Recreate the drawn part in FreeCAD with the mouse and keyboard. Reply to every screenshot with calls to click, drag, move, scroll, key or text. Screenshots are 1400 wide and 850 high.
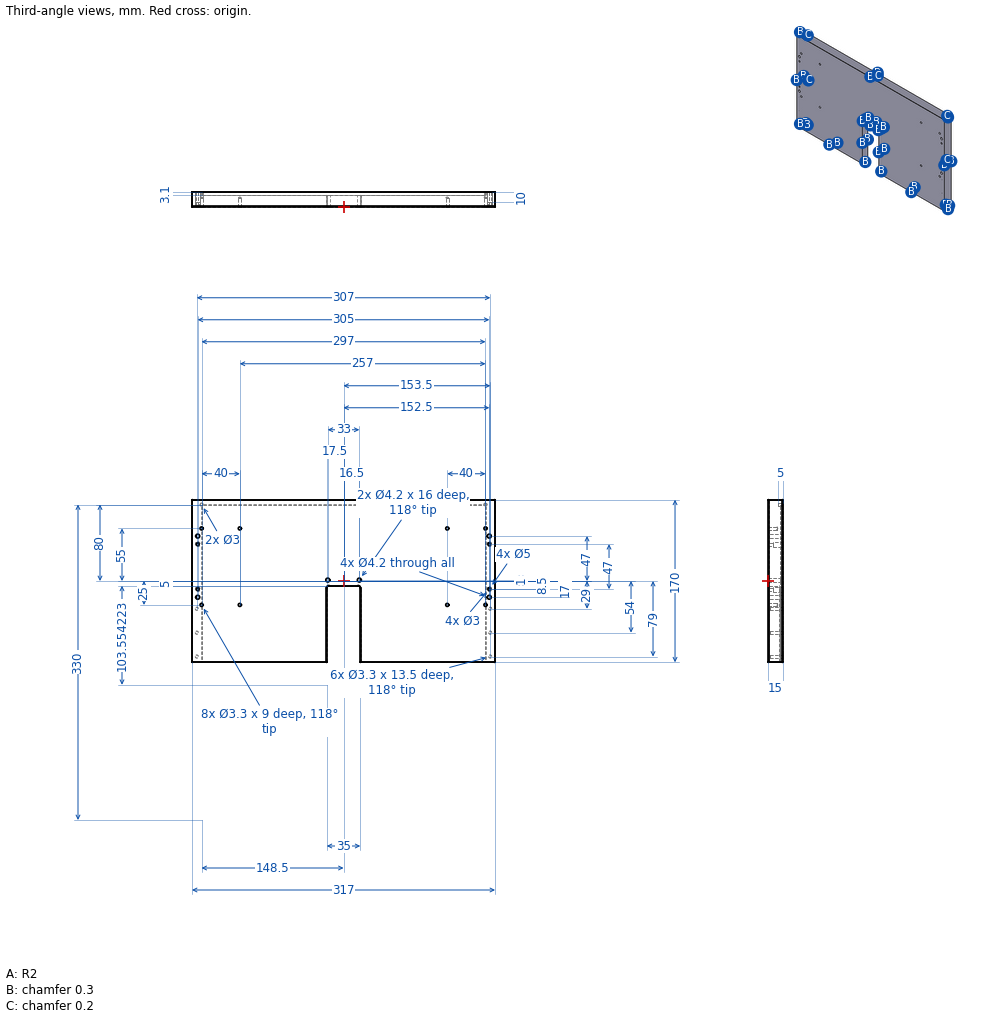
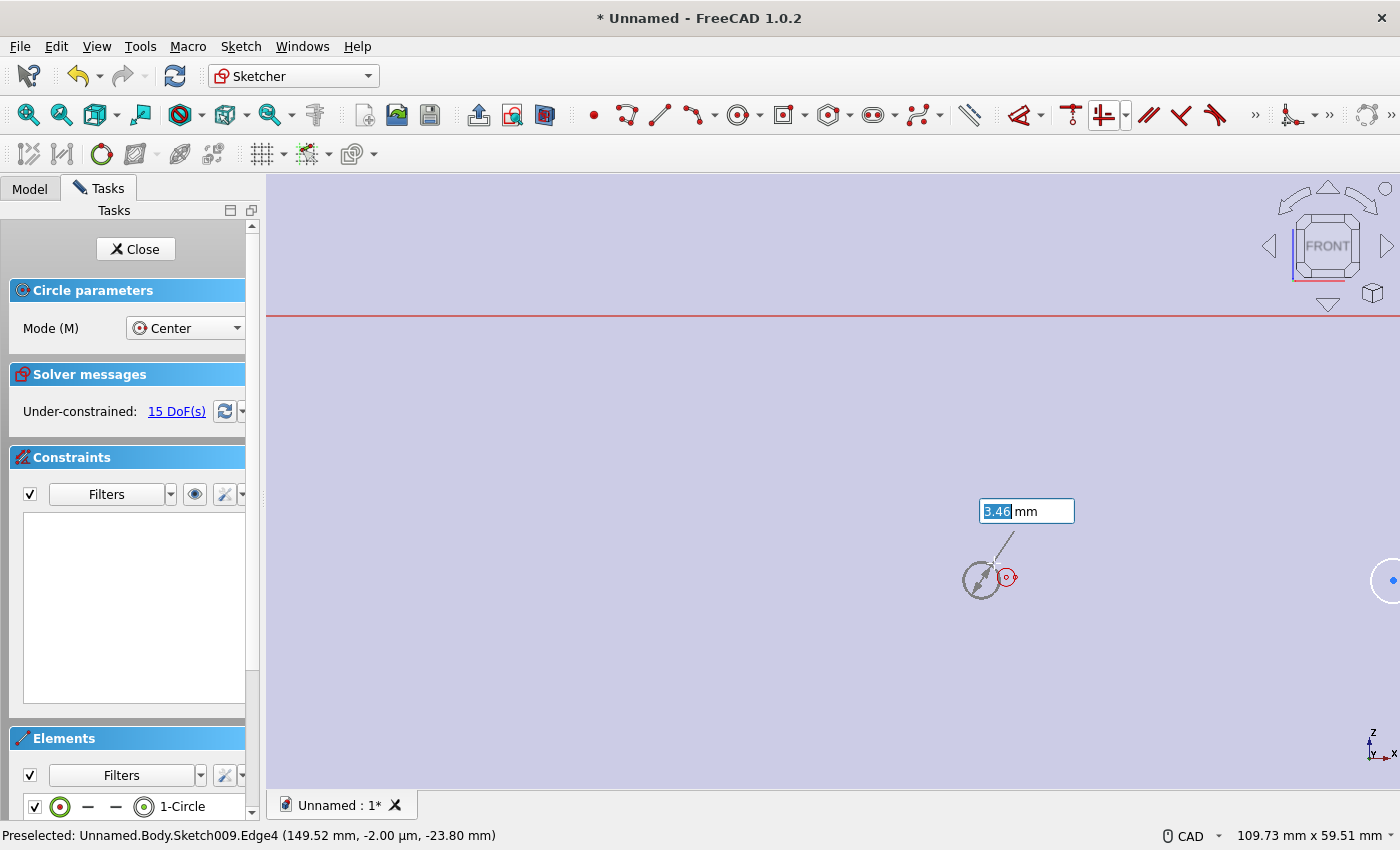
click(993, 563)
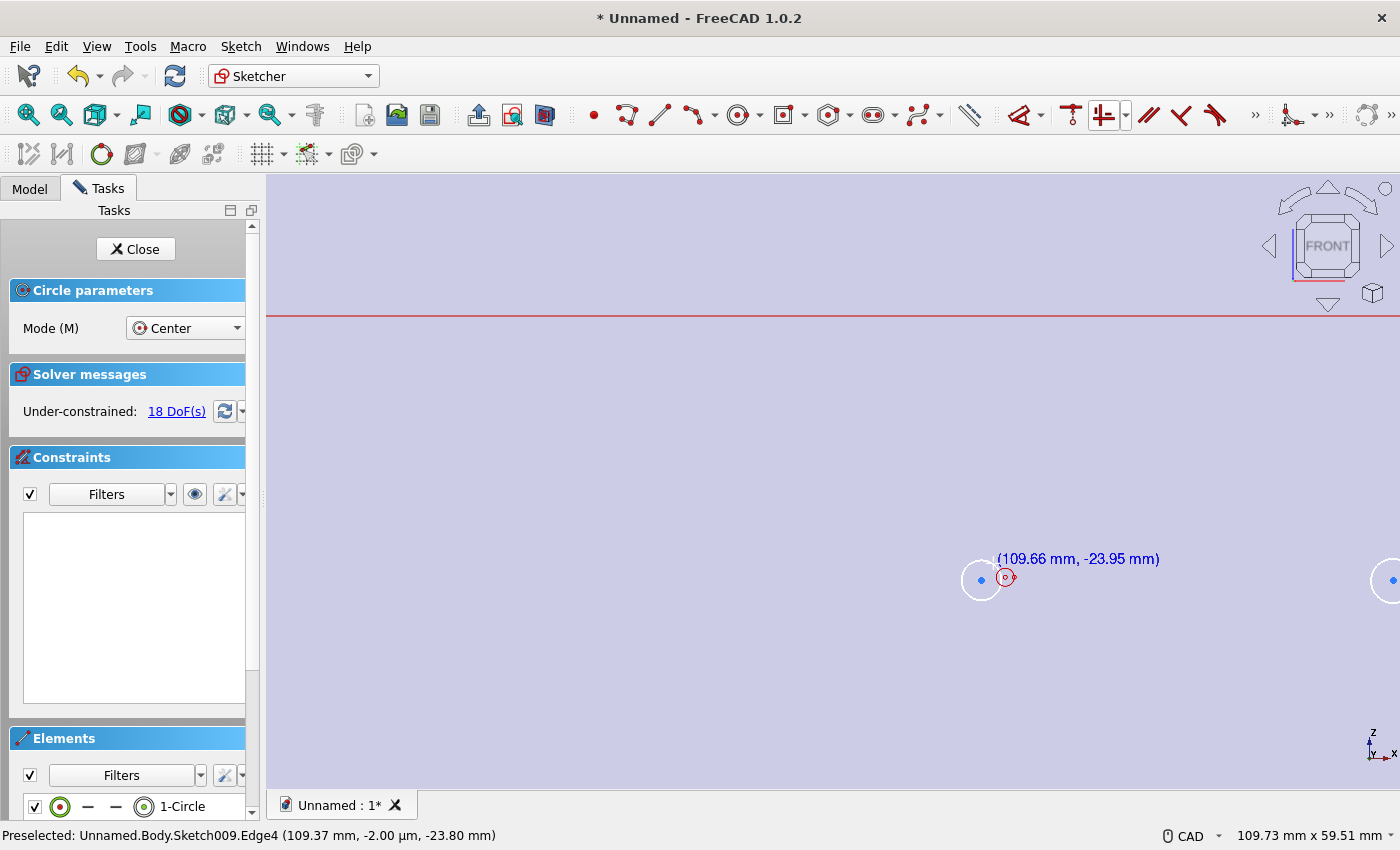
scroll(993, 562, down, 8)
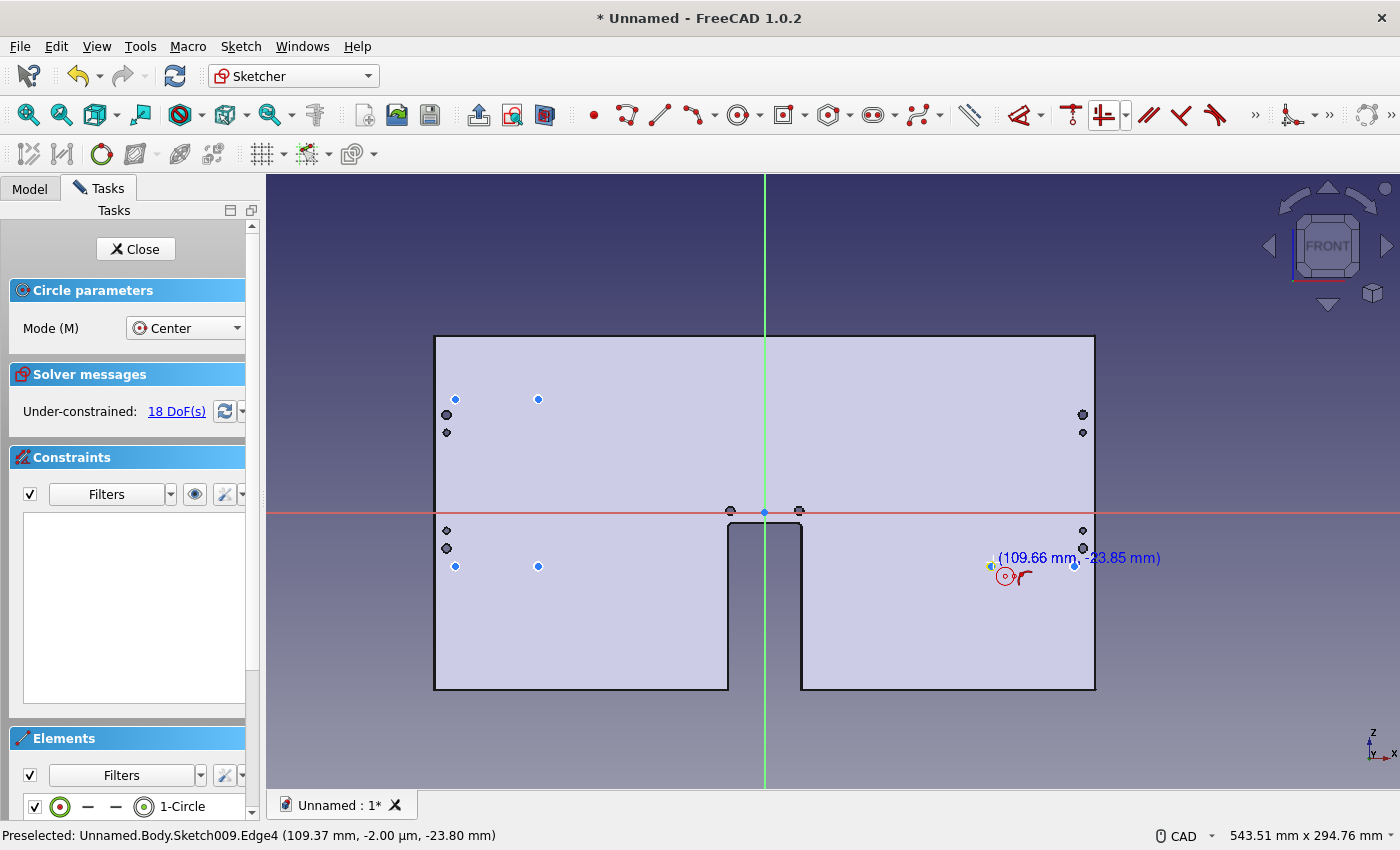
scroll(1075, 398, up, 10)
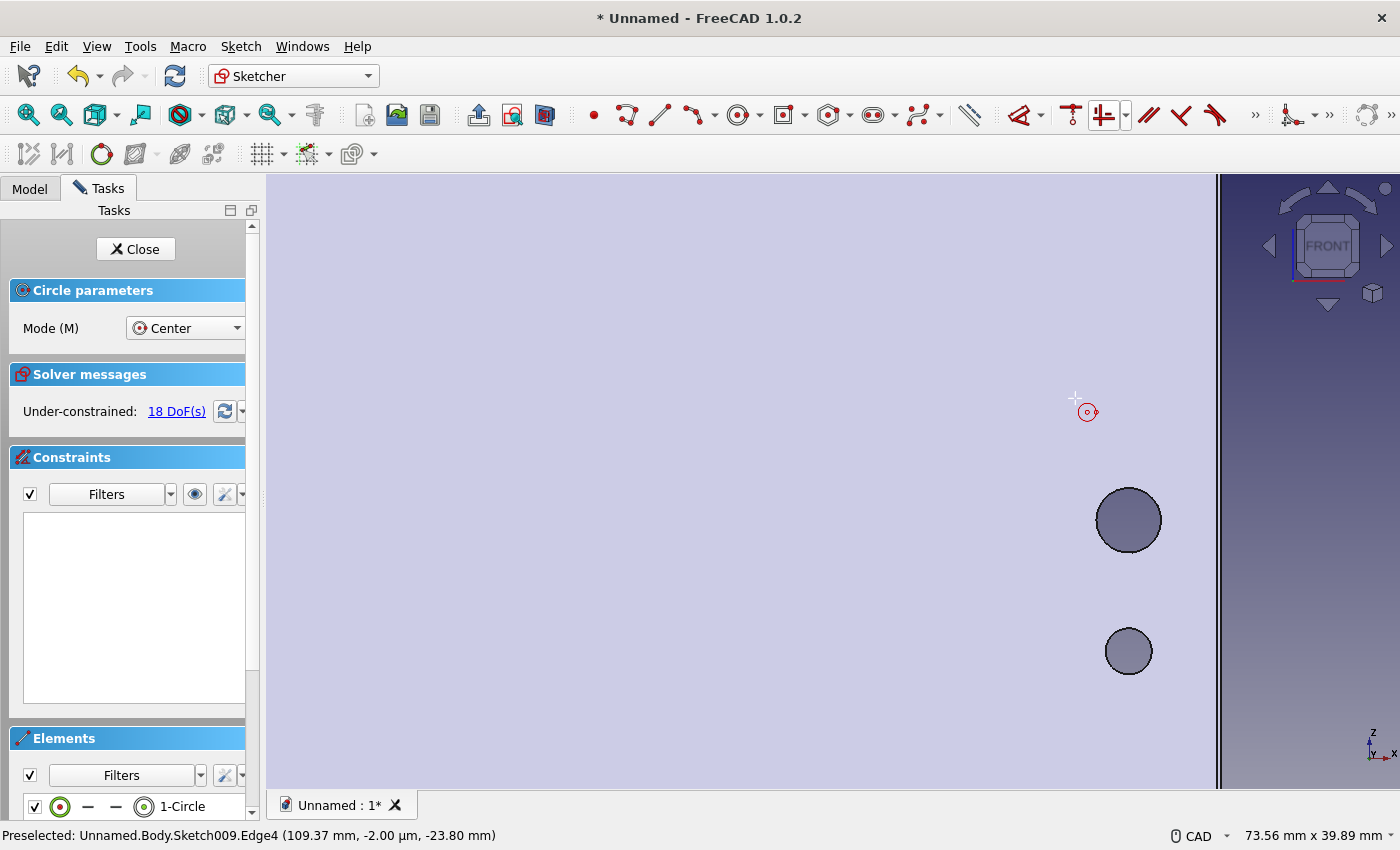
scroll(1075, 398, down, 10)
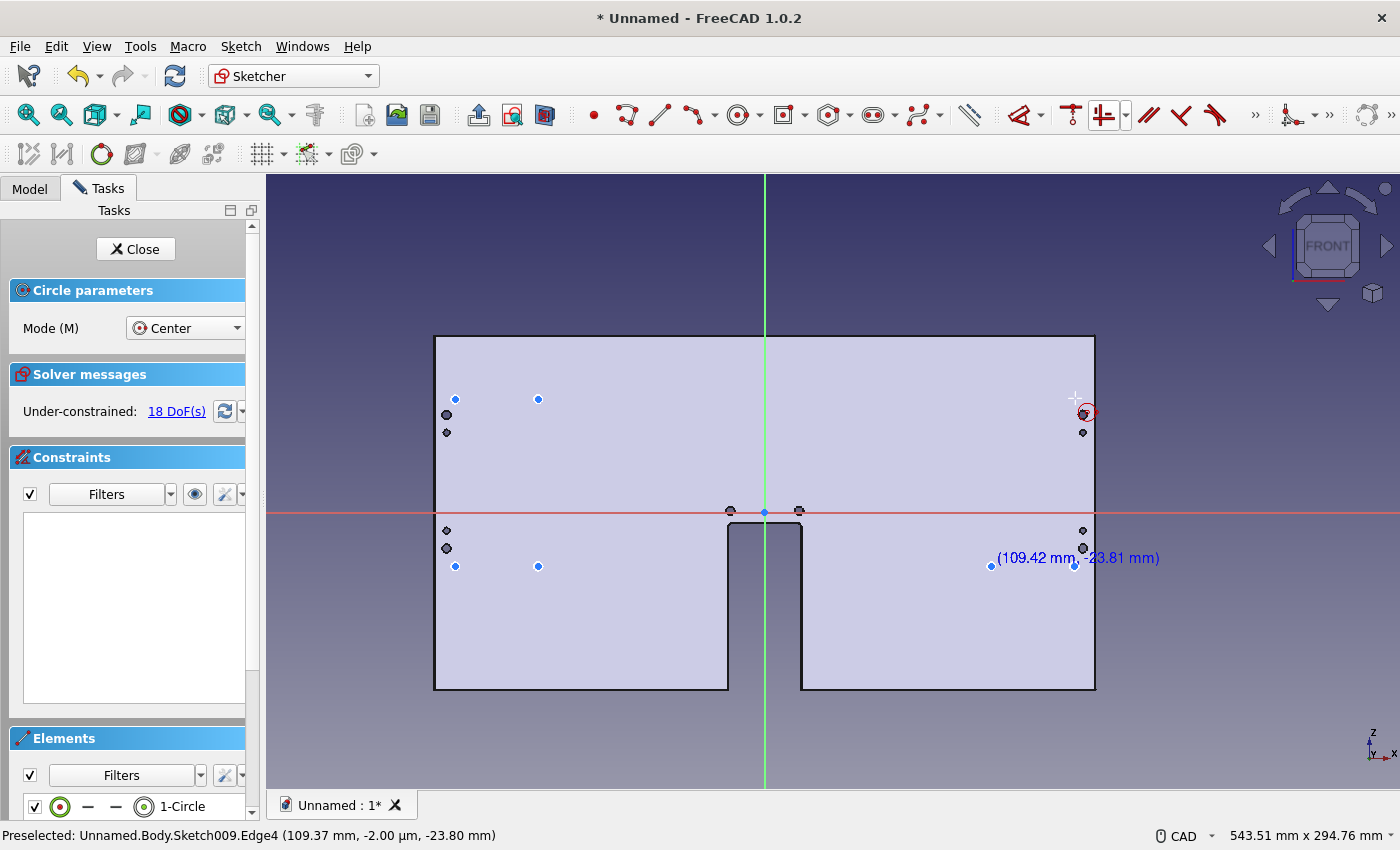
click(1075, 398)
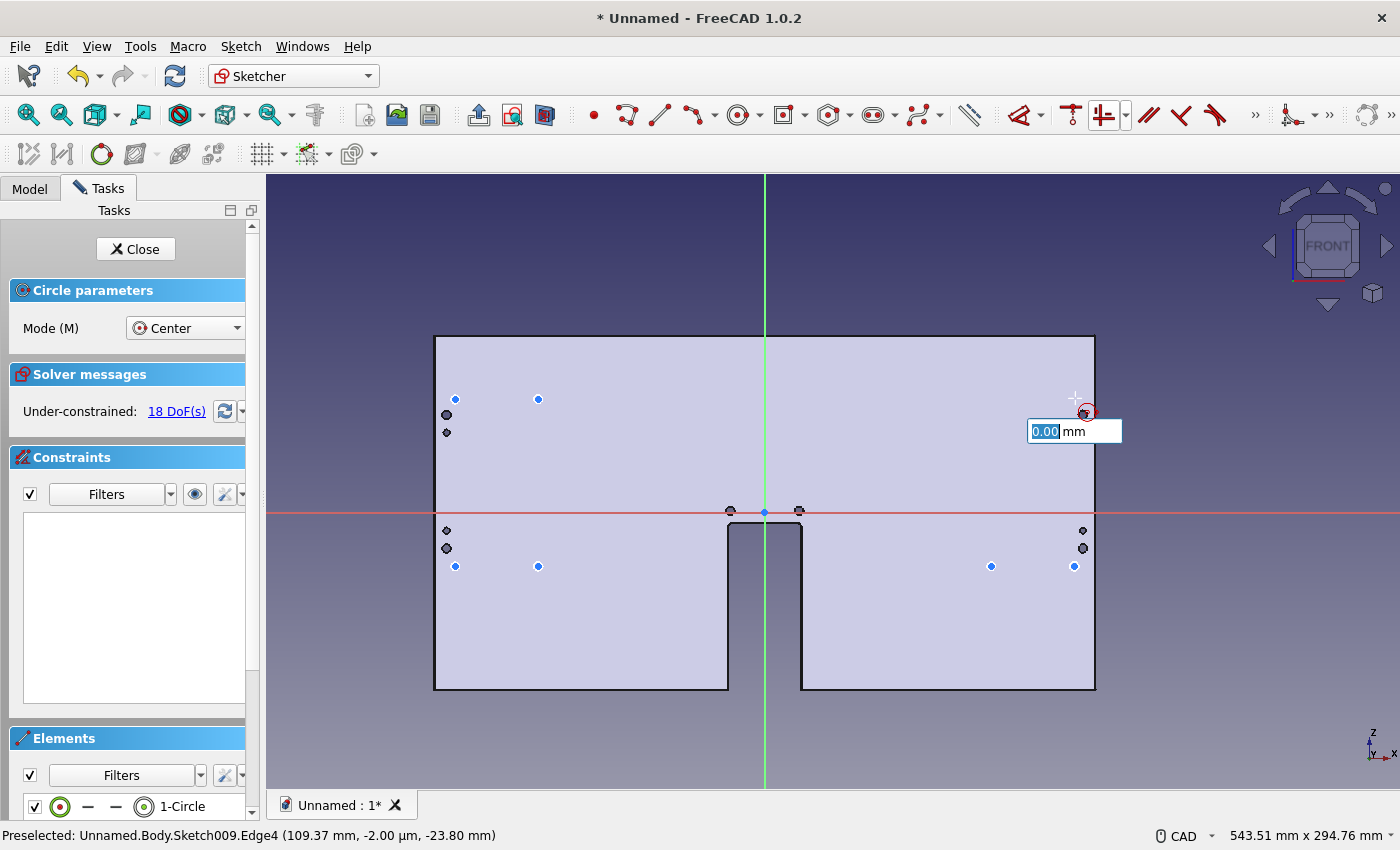
scroll(1077, 396, up, 8)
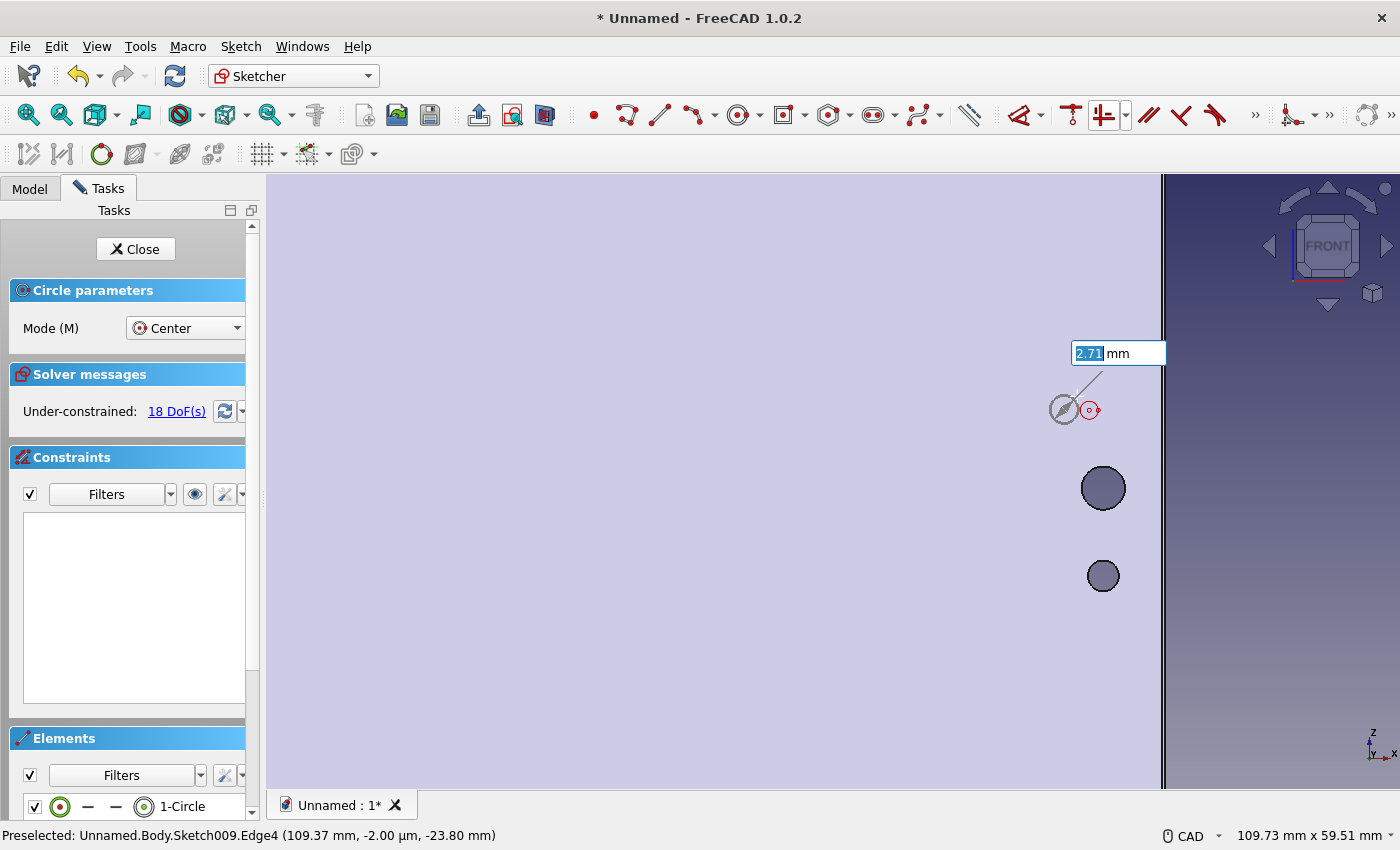
click(1074, 393)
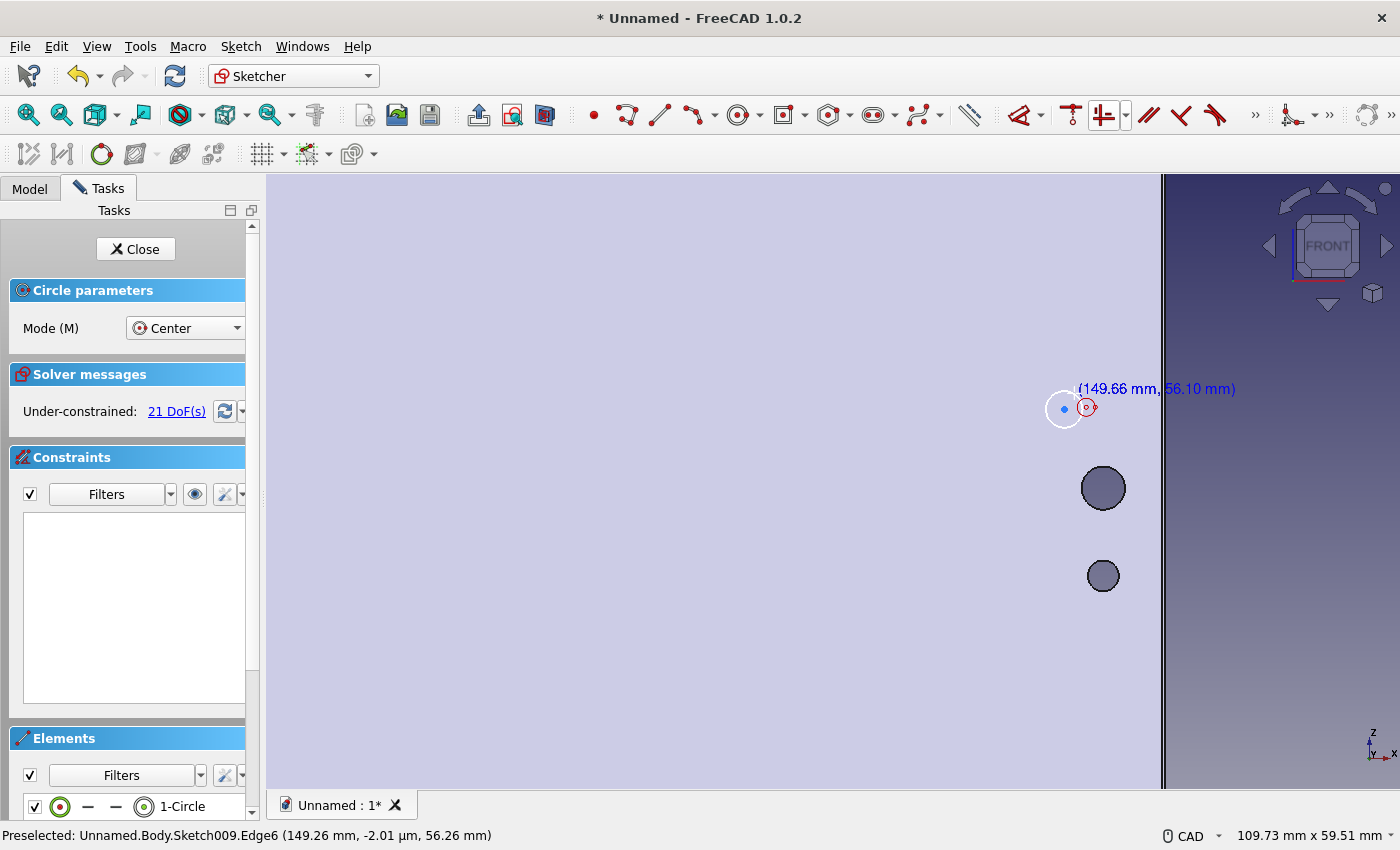
scroll(649, 405, up, 2)